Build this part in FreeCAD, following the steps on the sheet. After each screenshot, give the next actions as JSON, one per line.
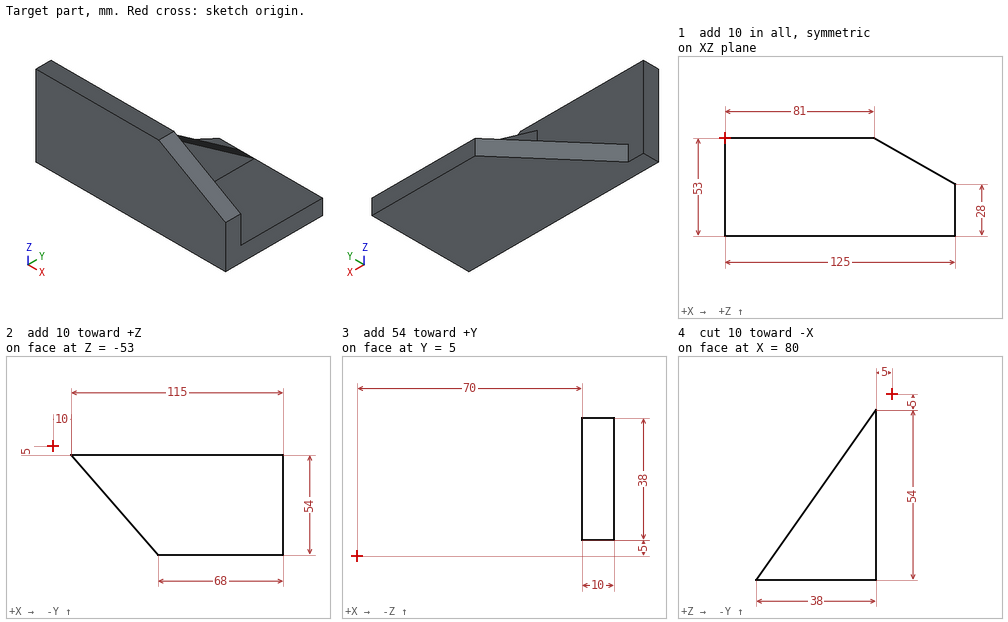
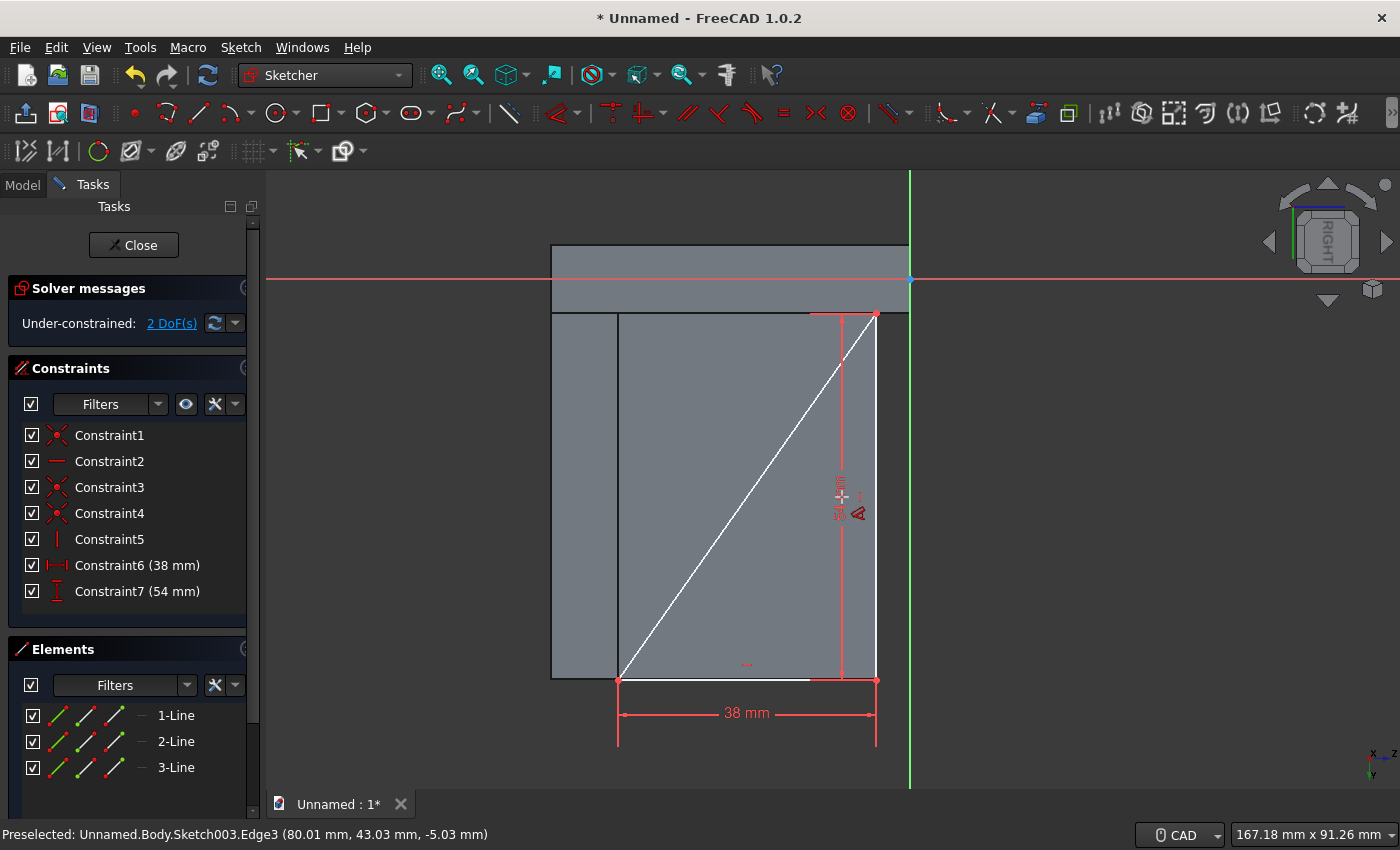
{"action": "left_click", "coordinate": [876, 314]}
{"action": "left_click", "coordinate": [893, 245]}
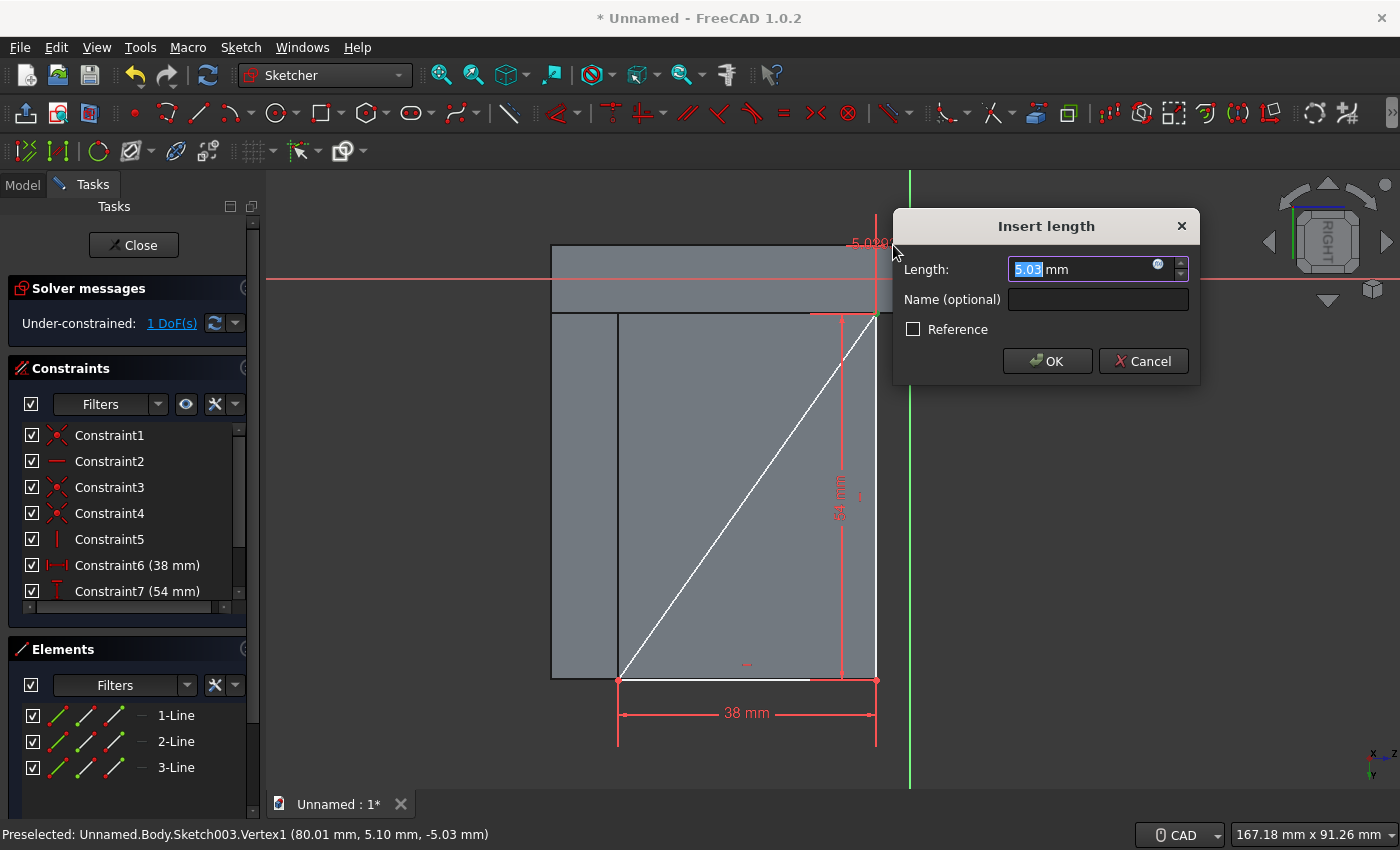
{"action": "type", "text": "5"}
{"action": "key", "text": "Return"}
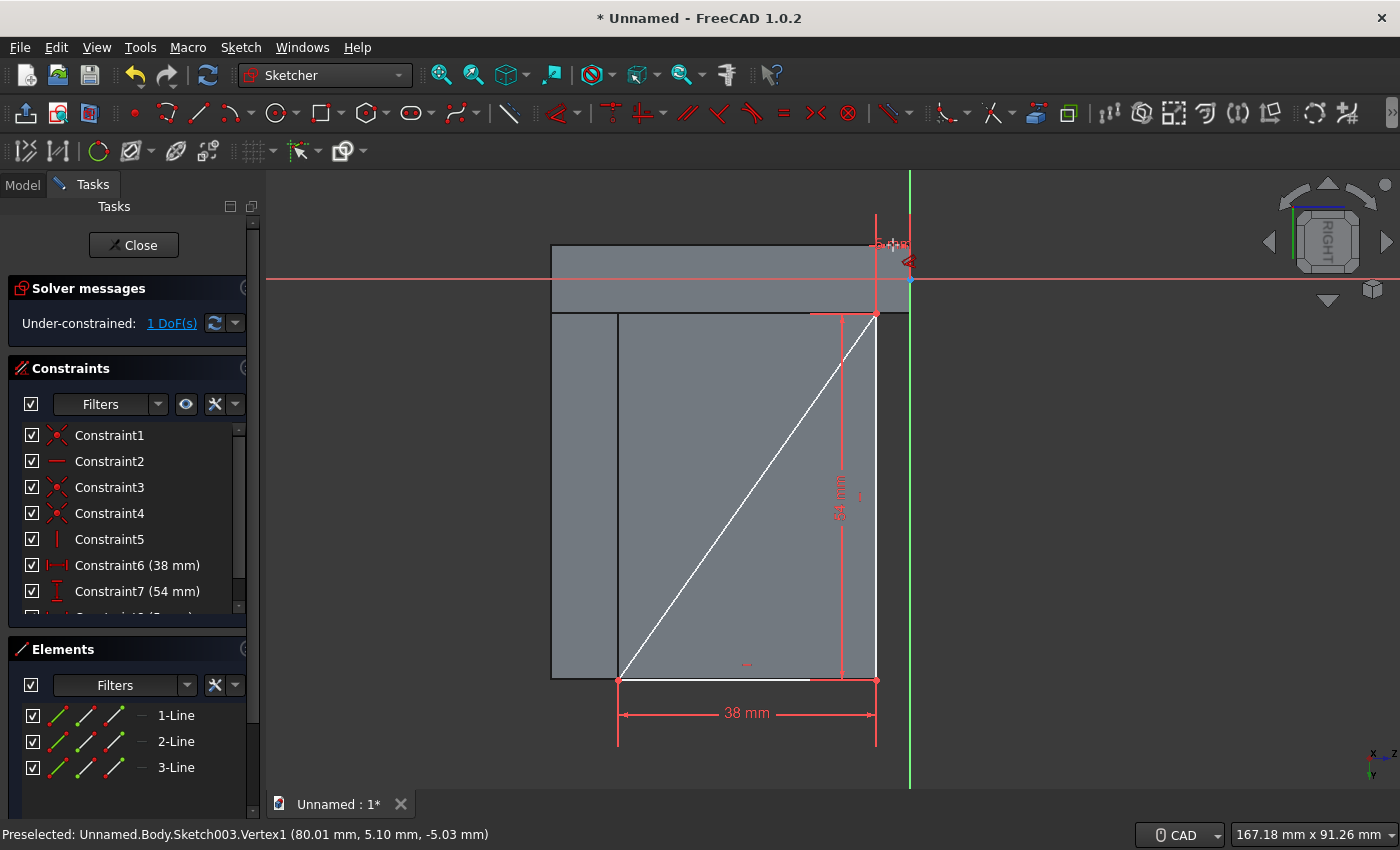
{"action": "left_click", "coordinate": [876, 314]}
{"action": "left_click", "coordinate": [944, 296]}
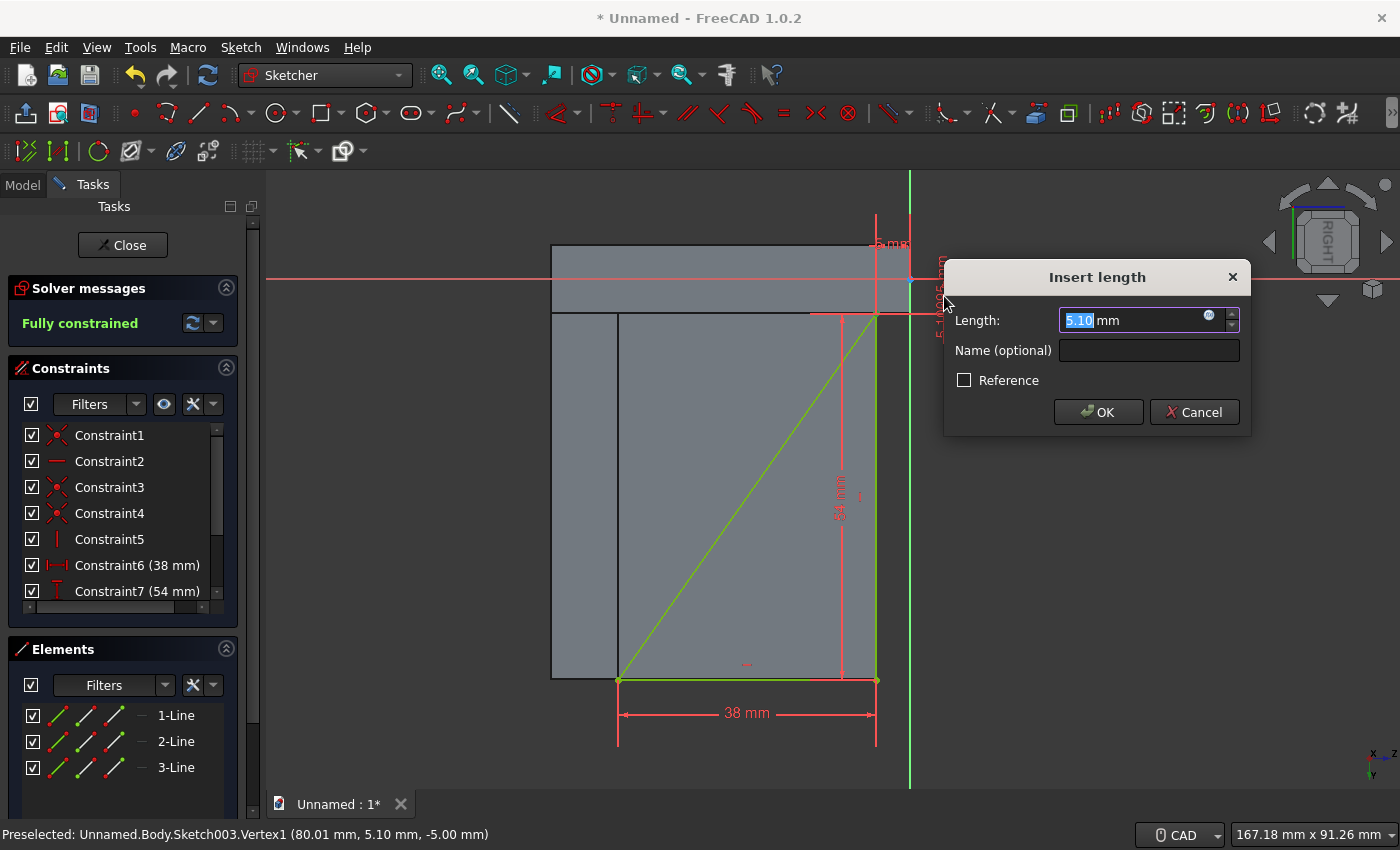
{"action": "type", "text": "5"}
{"action": "key", "text": "Return"}
{"action": "key", "text": "Escape"}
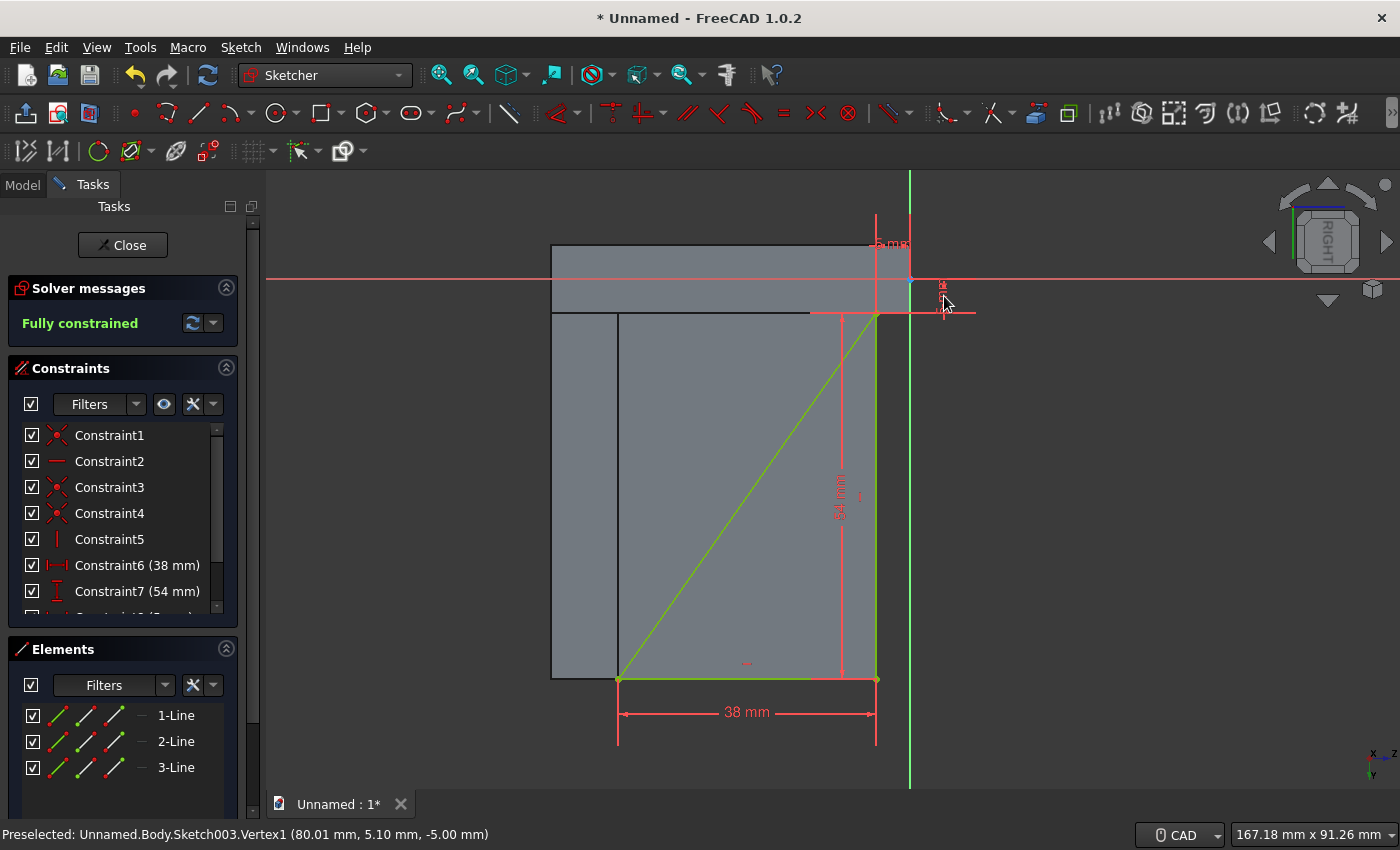
{"action": "left_click", "coordinate": [123, 245]}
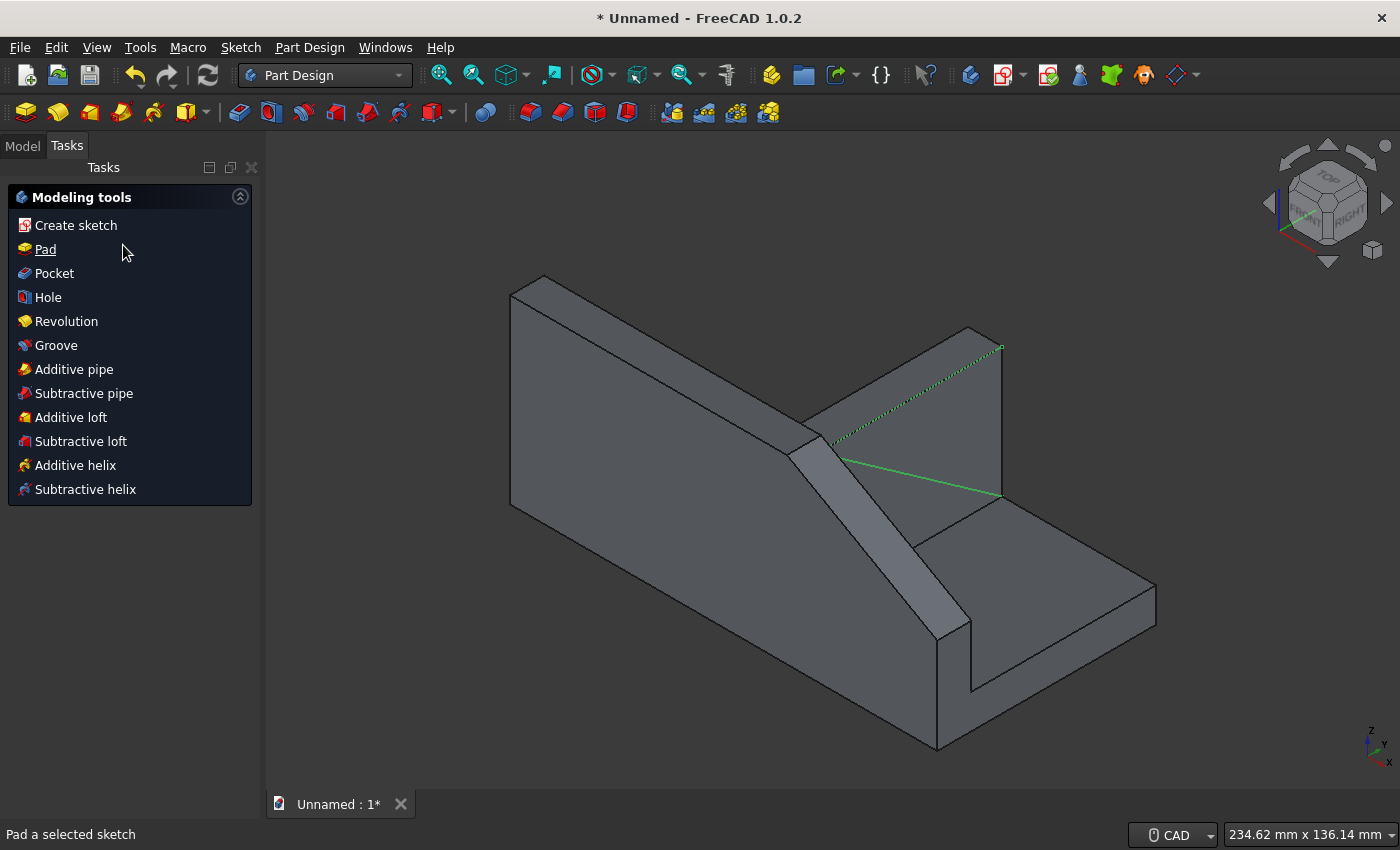
{"action": "left_click", "coordinate": [240, 112]}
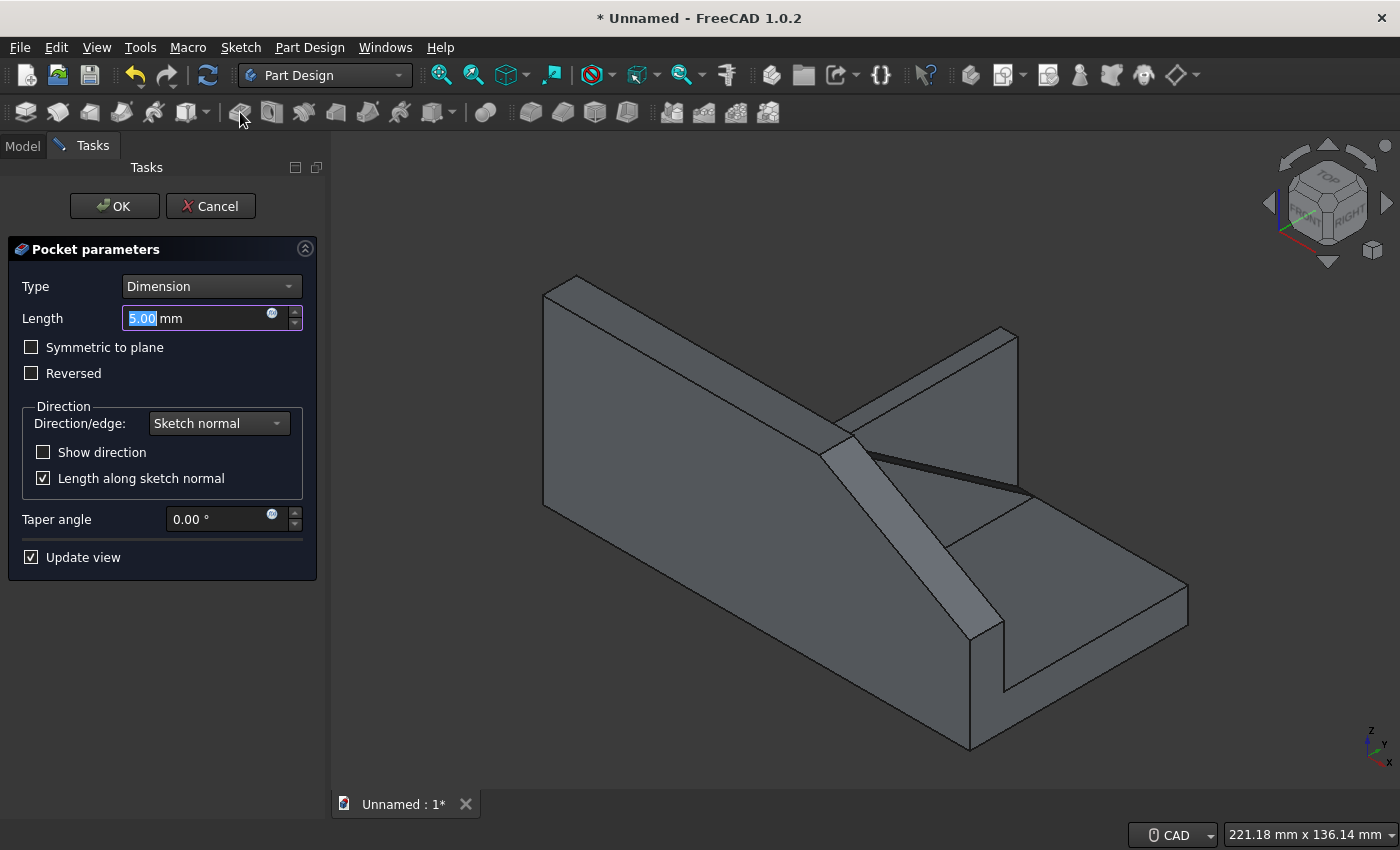
{"action": "type", "text": "10"}
{"action": "key", "text": "Tab"}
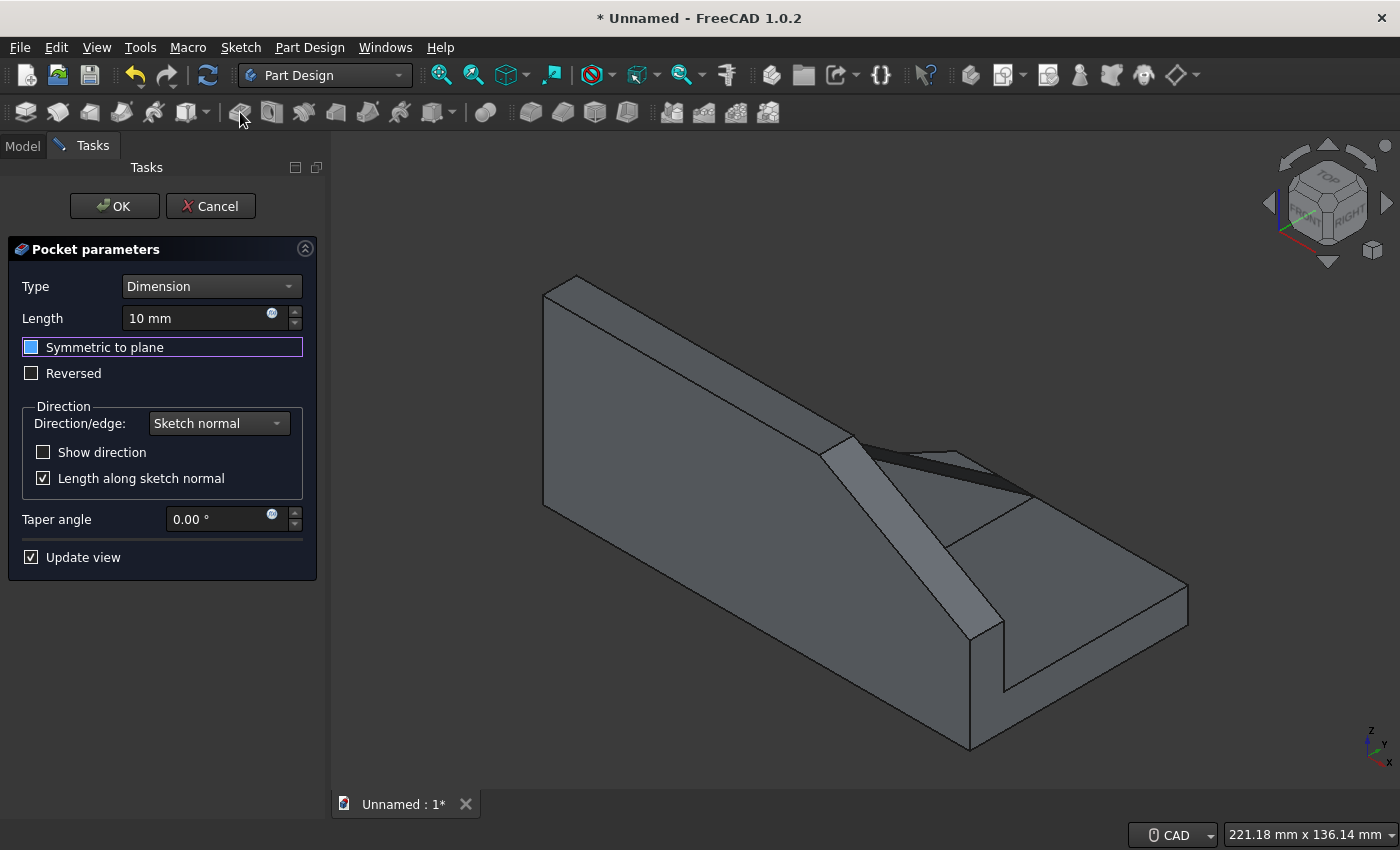
{"action": "left_click", "coordinate": [115, 206]}